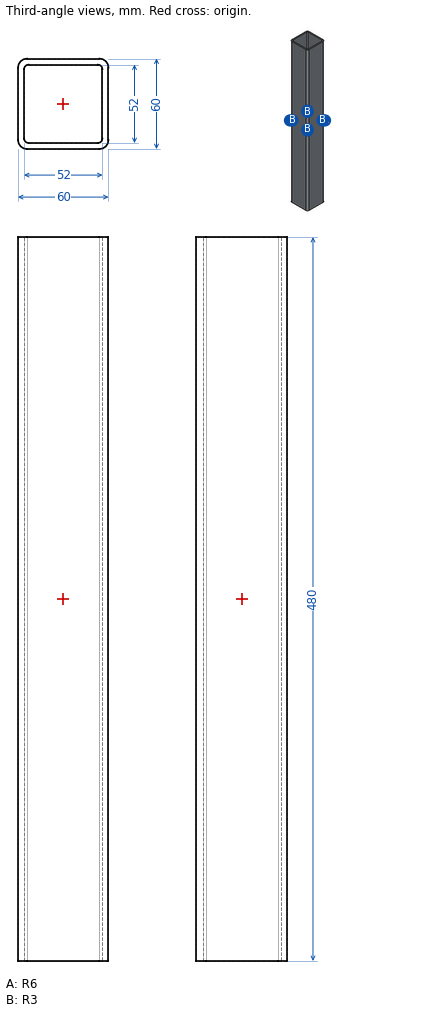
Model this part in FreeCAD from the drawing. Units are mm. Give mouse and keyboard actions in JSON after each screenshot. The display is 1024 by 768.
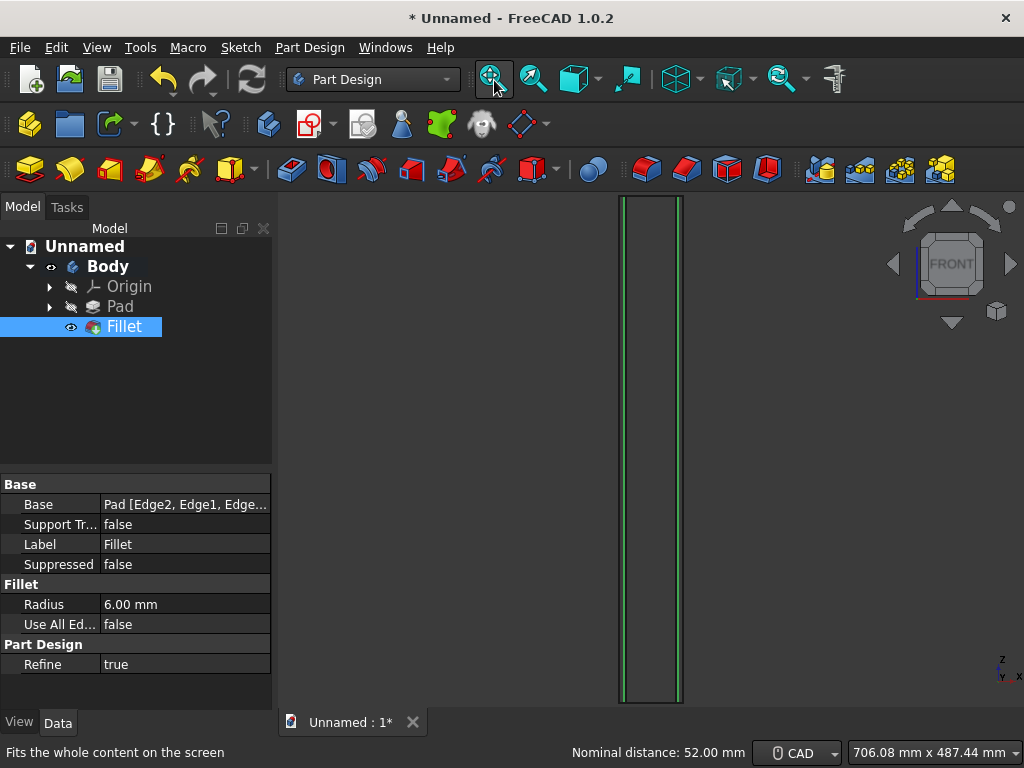
{"action": "key", "text": "3"}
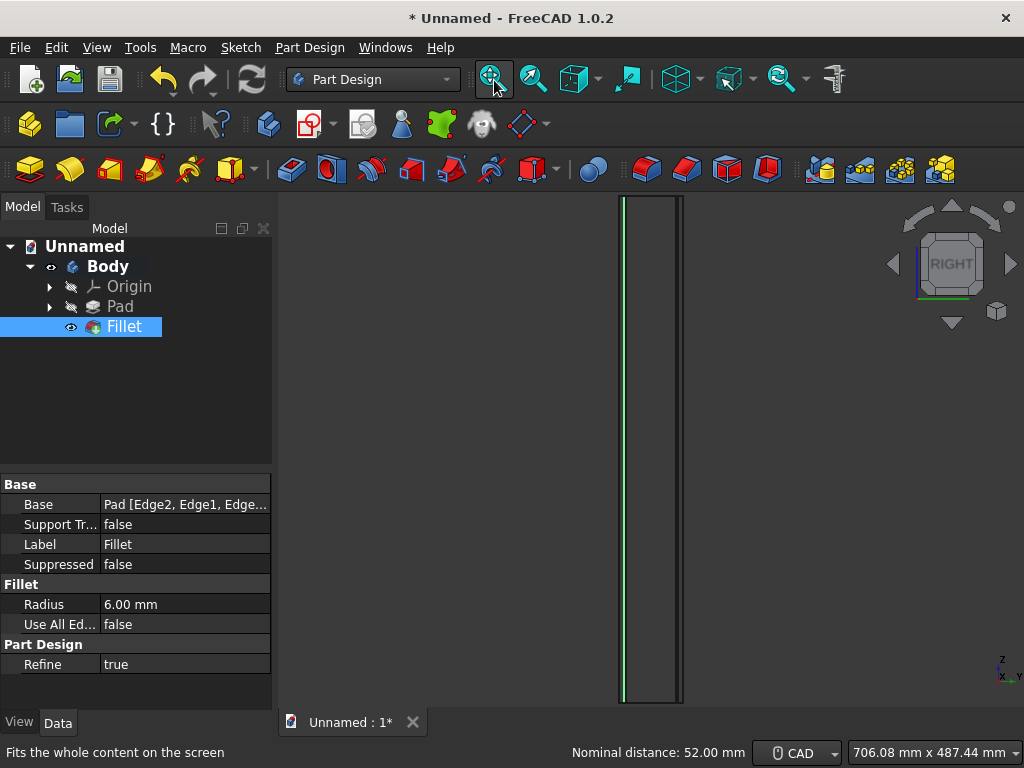
{"action": "scroll", "coordinate": [678, 448], "scroll_direction": "up", "scroll_amount": 6}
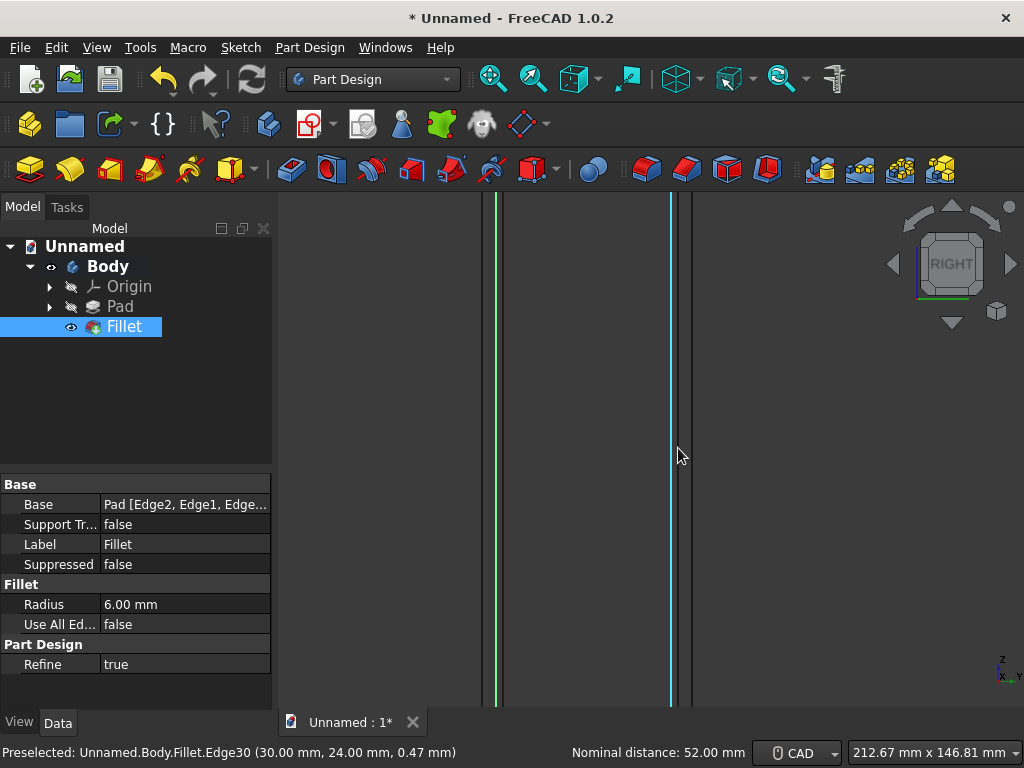
{"action": "left_click", "coordinate": [678, 451], "text": "ctrl"}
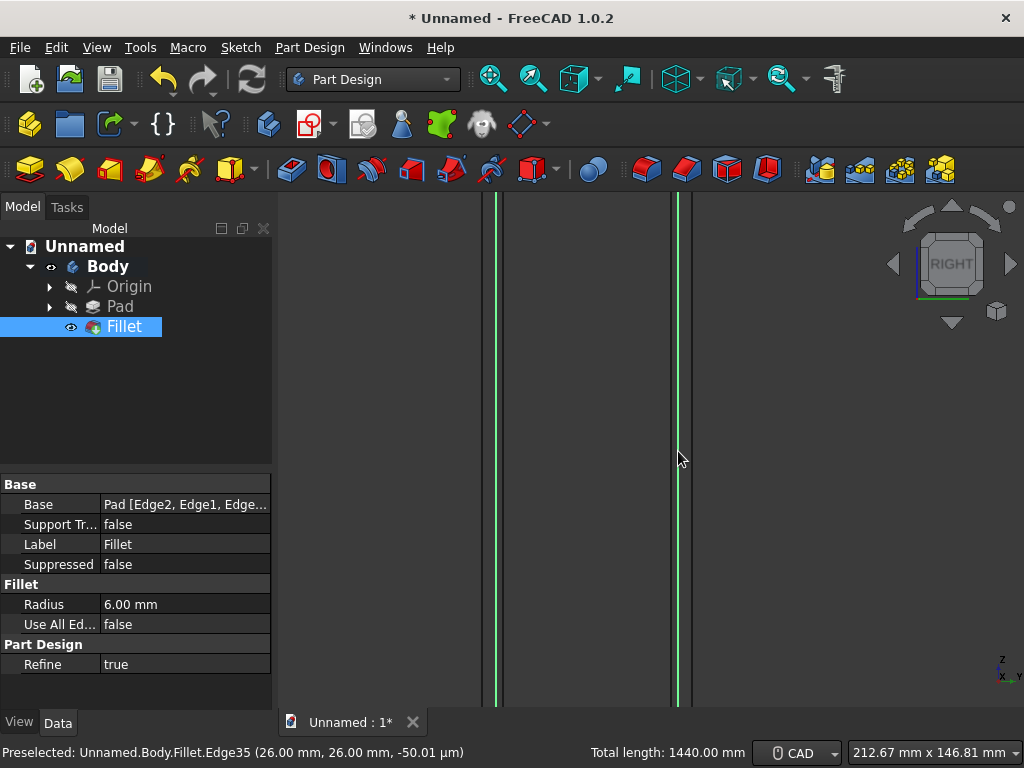
{"action": "left_click", "coordinate": [494, 80]}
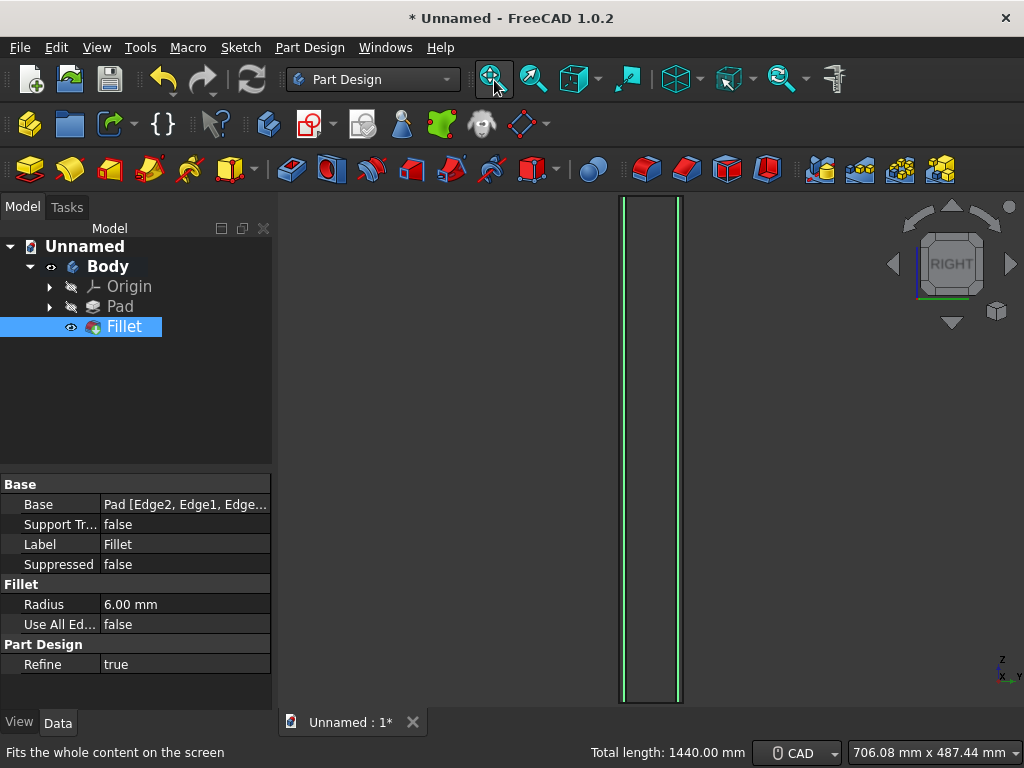
{"action": "key", "text": "5"}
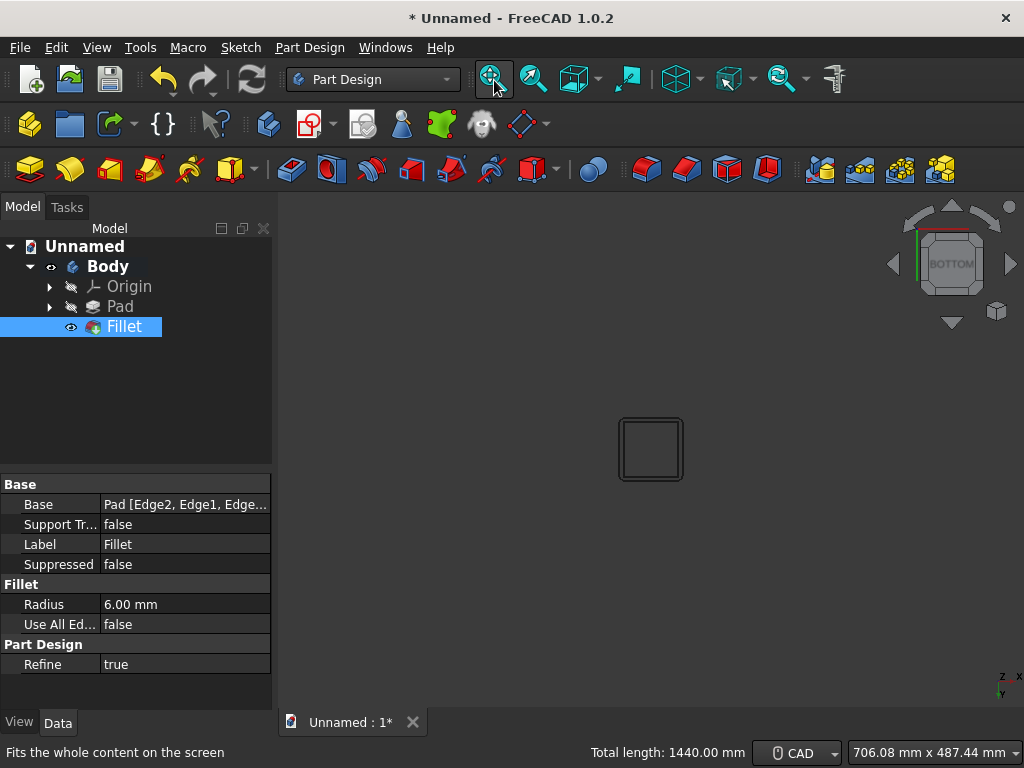
{"action": "left_click", "coordinate": [494, 80]}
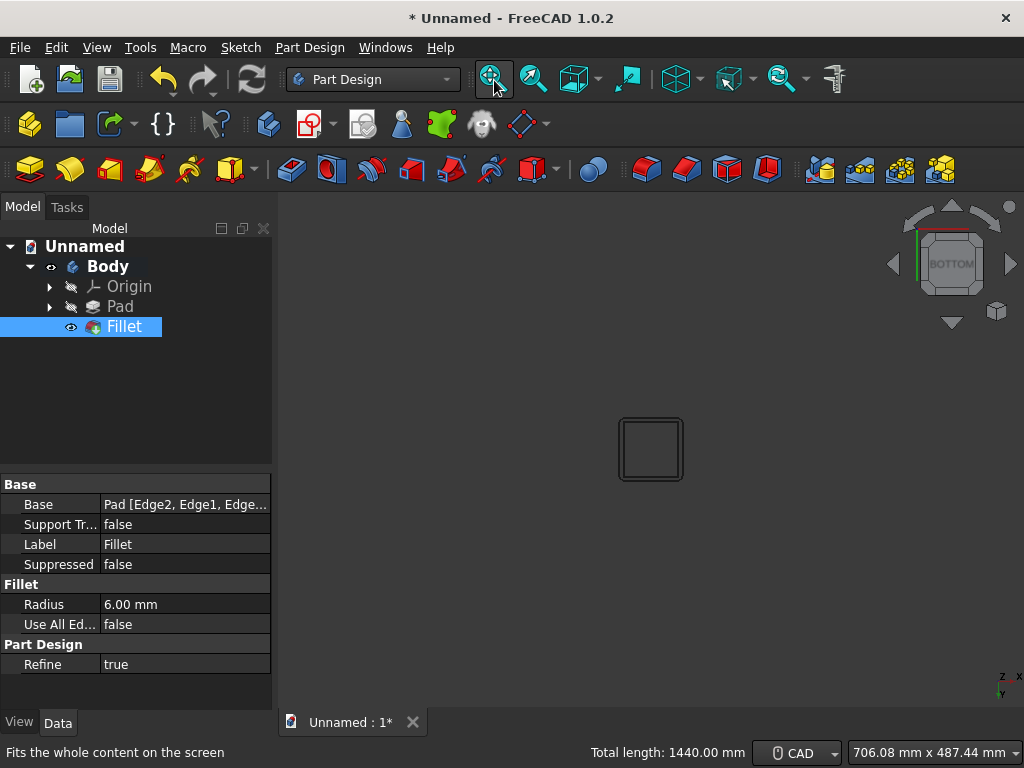
{"action": "scroll", "coordinate": [624, 476], "scroll_direction": "up", "scroll_amount": 6}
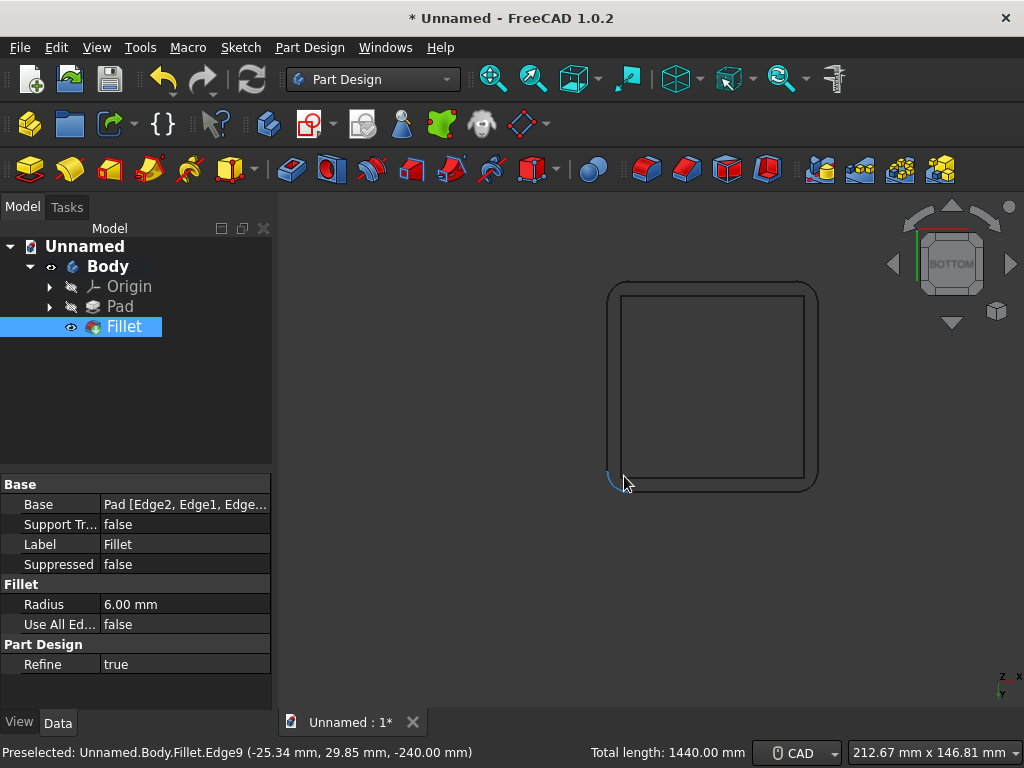
{"action": "left_click", "coordinate": [494, 80]}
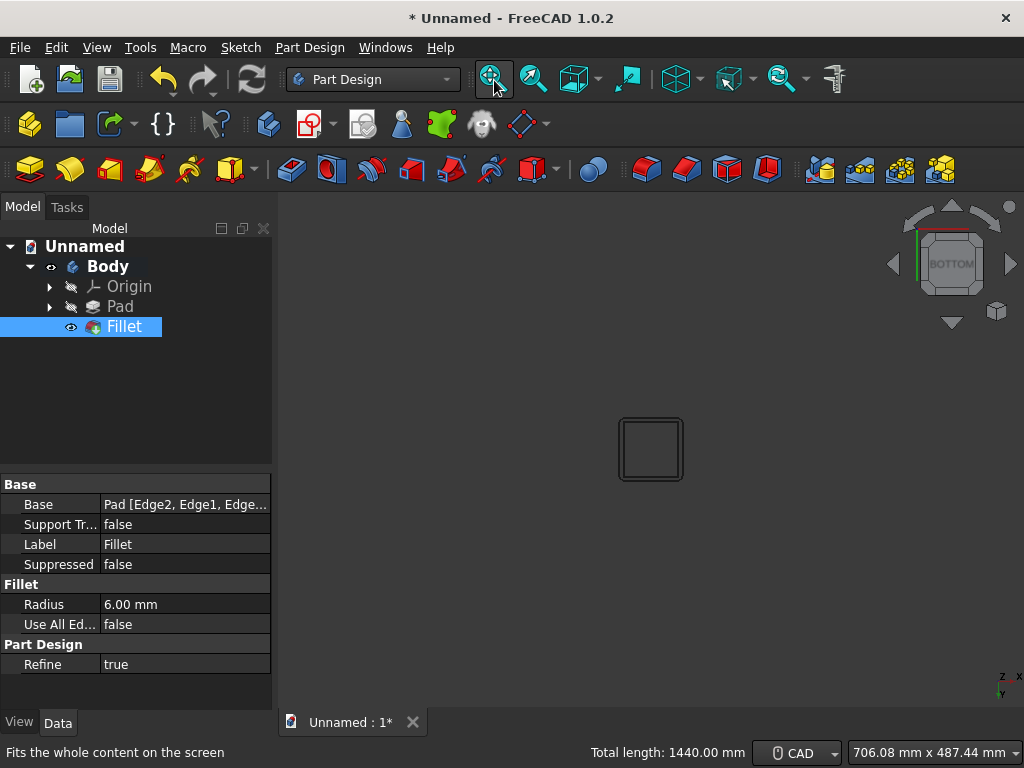
{"action": "key", "text": "4"}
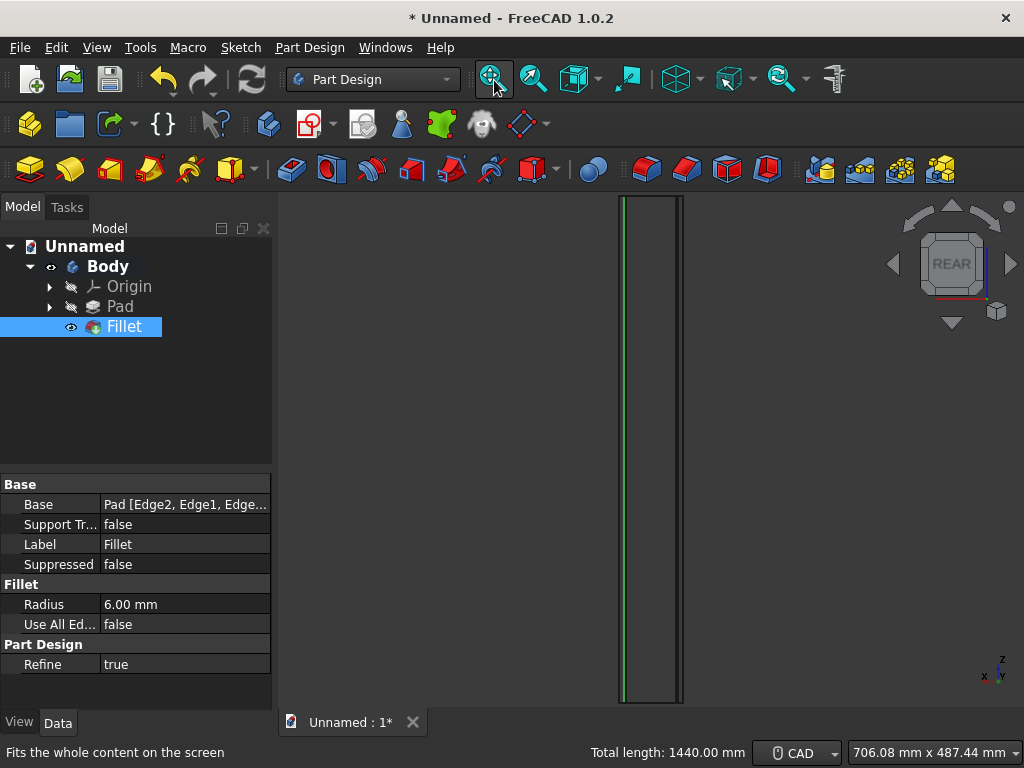
{"action": "scroll", "coordinate": [678, 449], "scroll_direction": "up", "scroll_amount": 6}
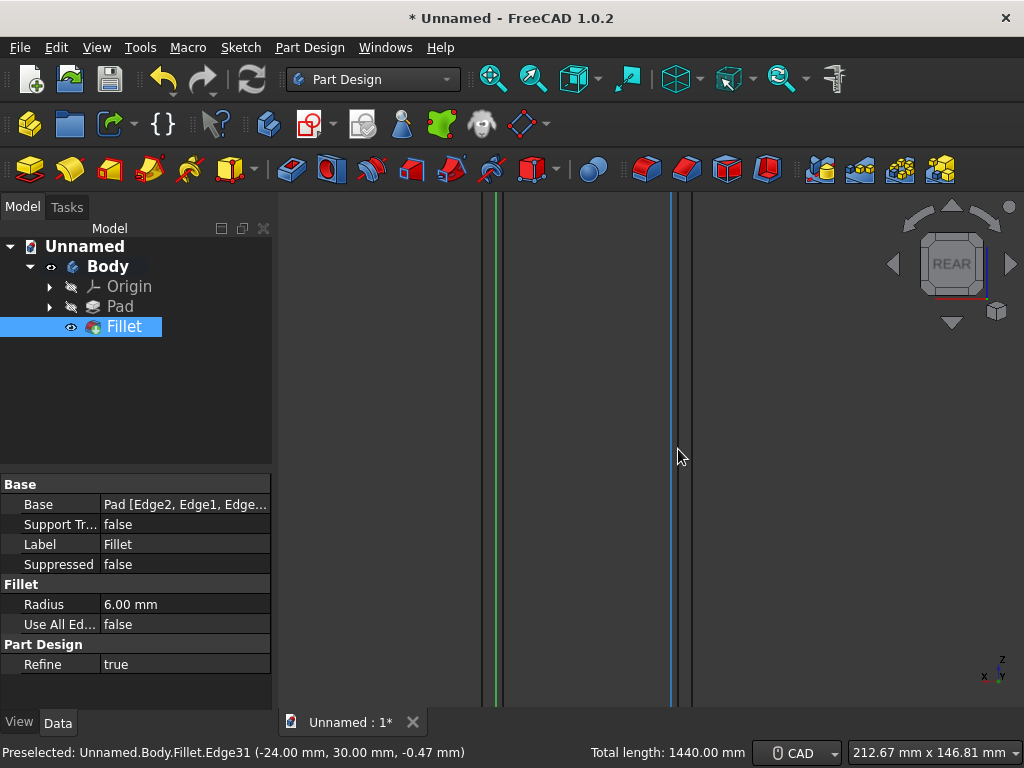
{"action": "left_click", "coordinate": [678, 449], "text": "ctrl"}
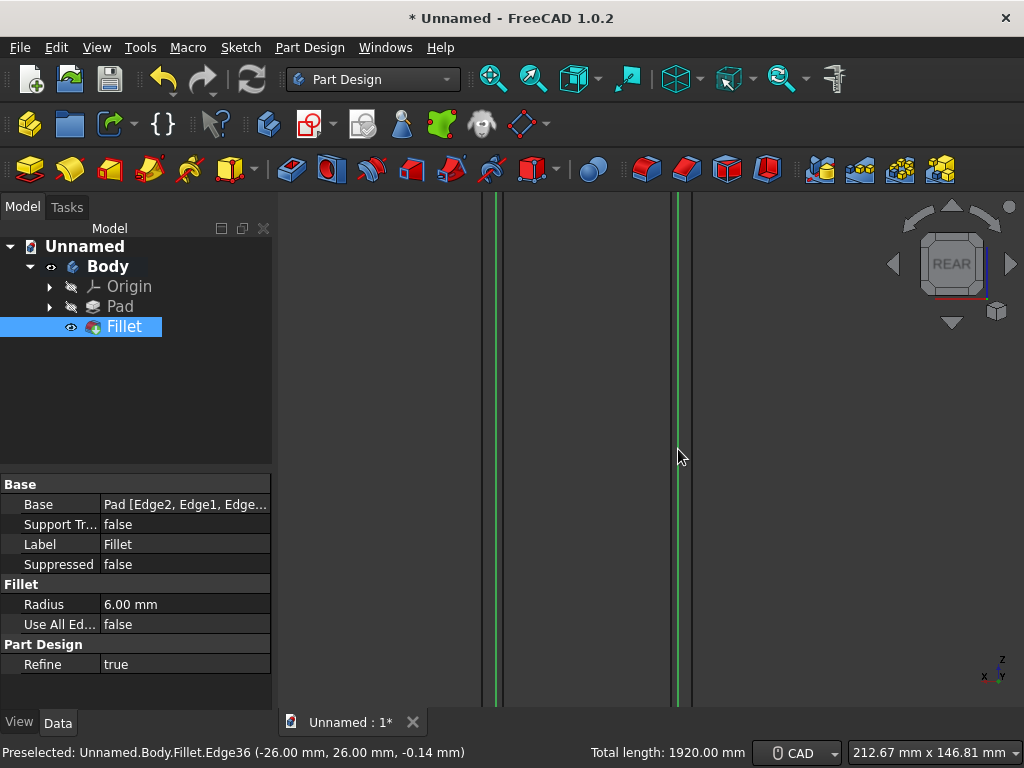
{"action": "key", "text": "v 1"}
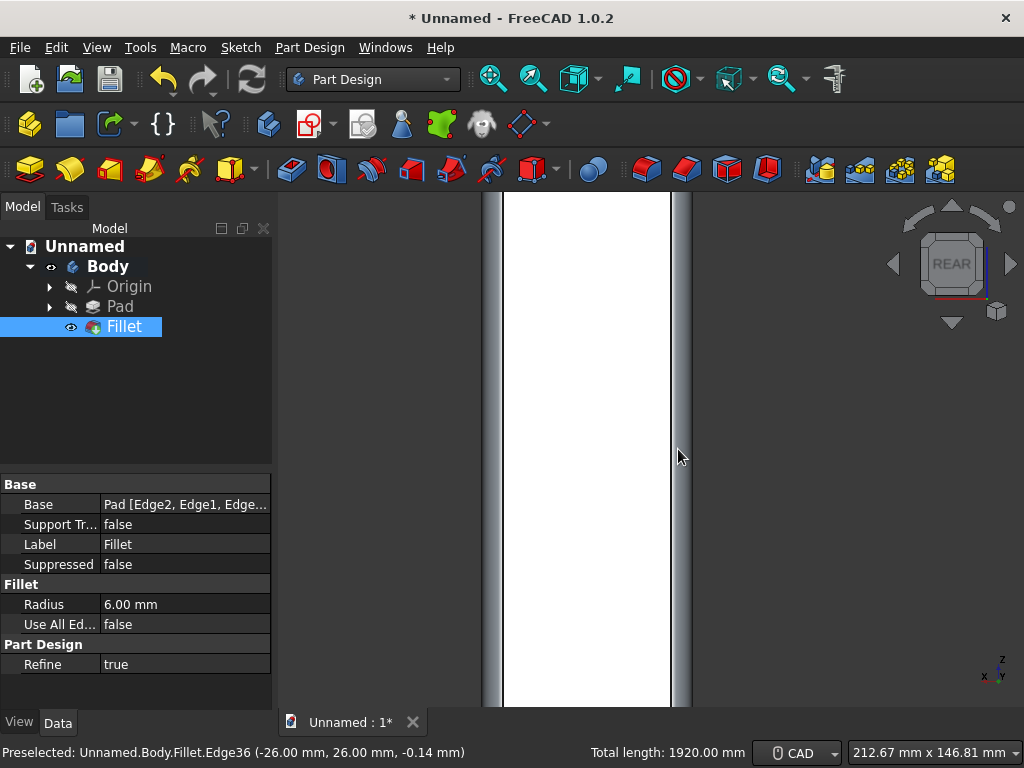
{"action": "left_click", "coordinate": [648, 170]}